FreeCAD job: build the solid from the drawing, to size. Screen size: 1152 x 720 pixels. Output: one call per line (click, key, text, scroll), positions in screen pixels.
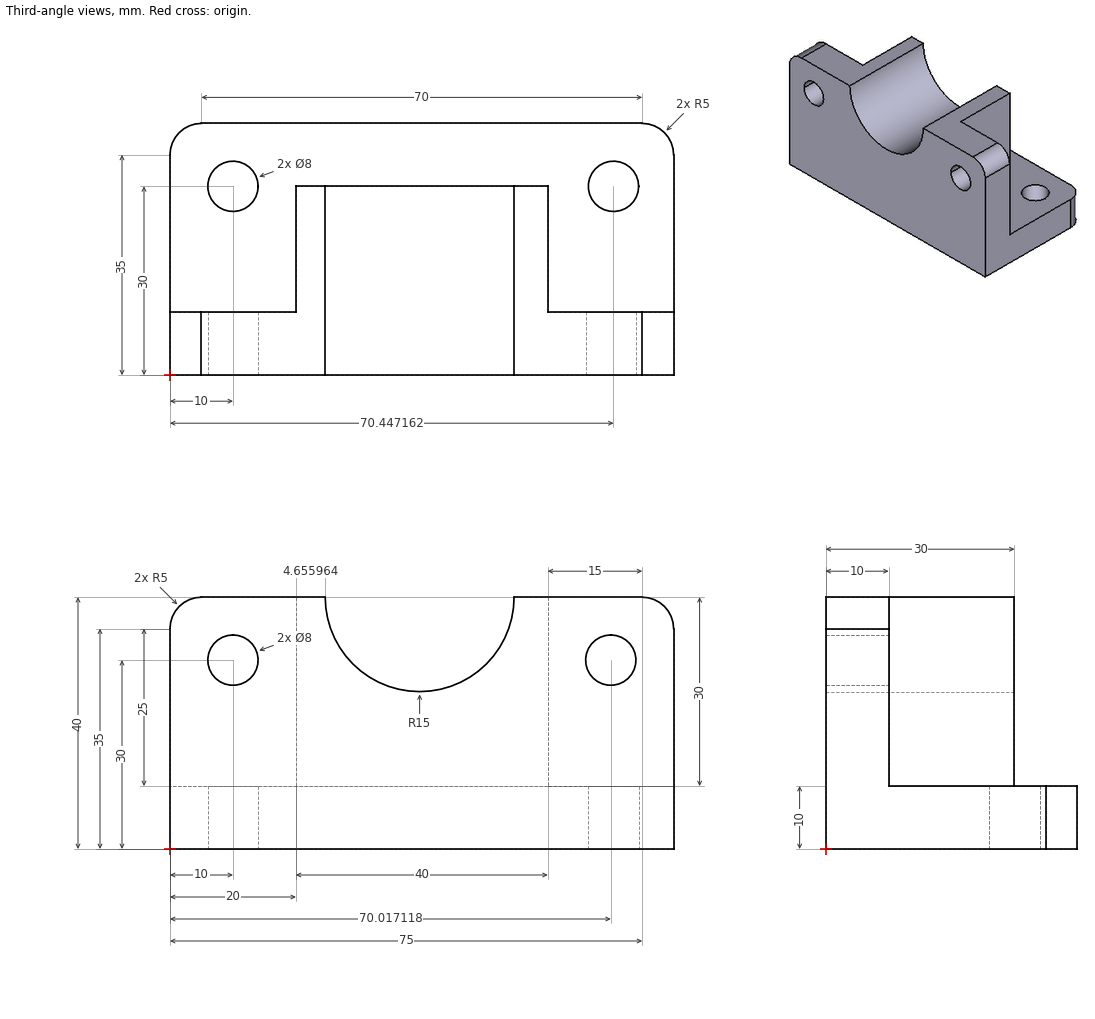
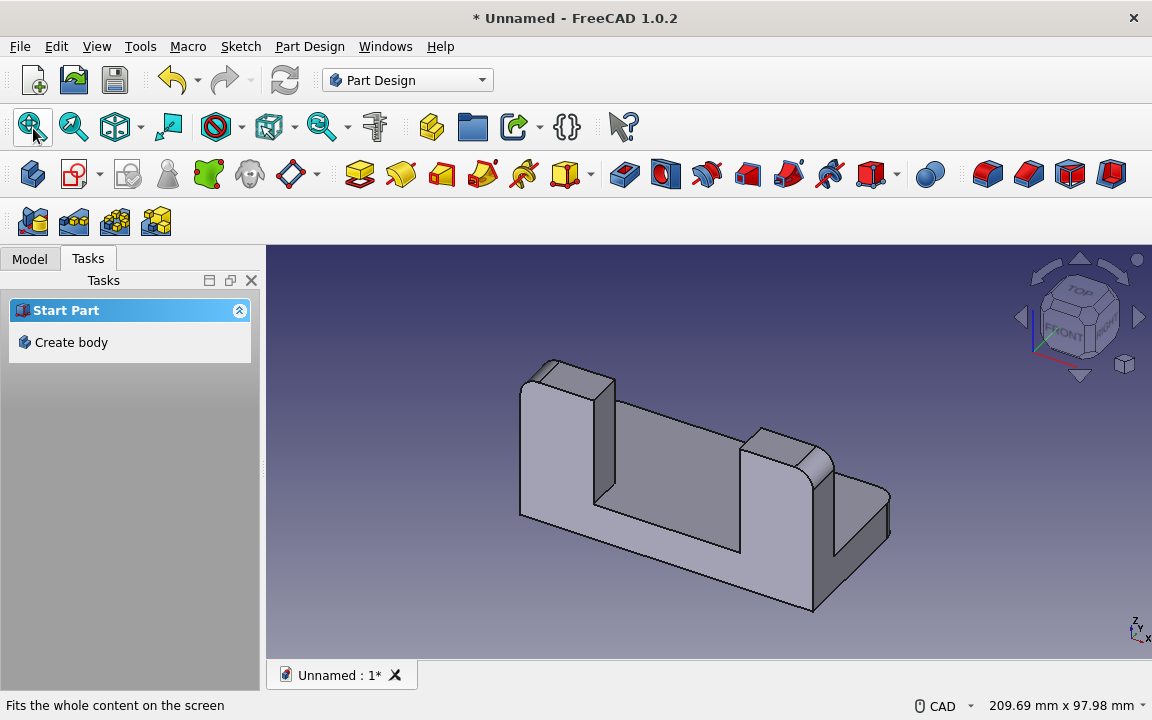
click(541, 412)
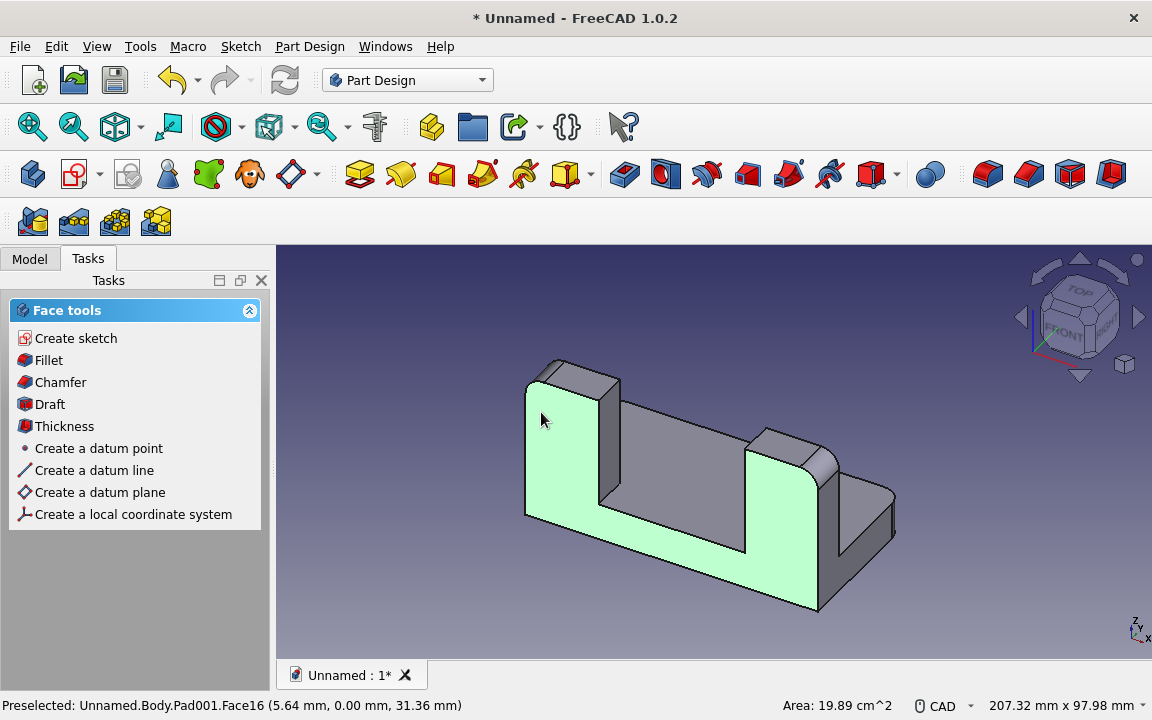
click(74, 174)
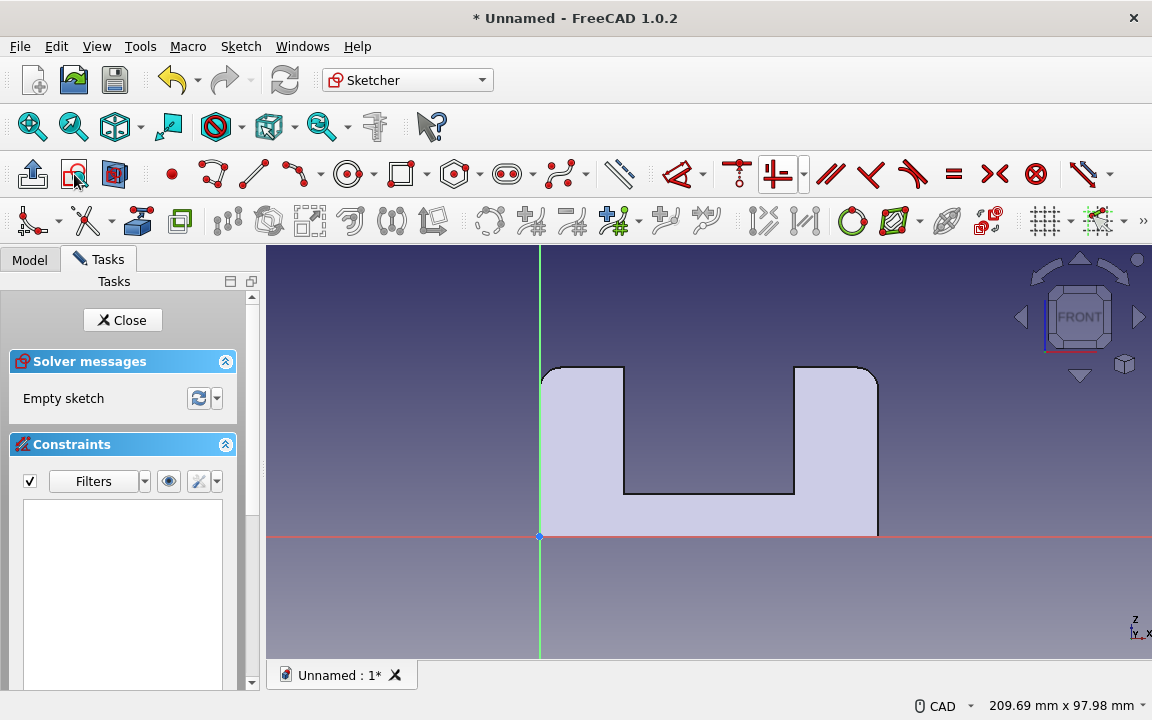
scroll(720, 452, up, 2)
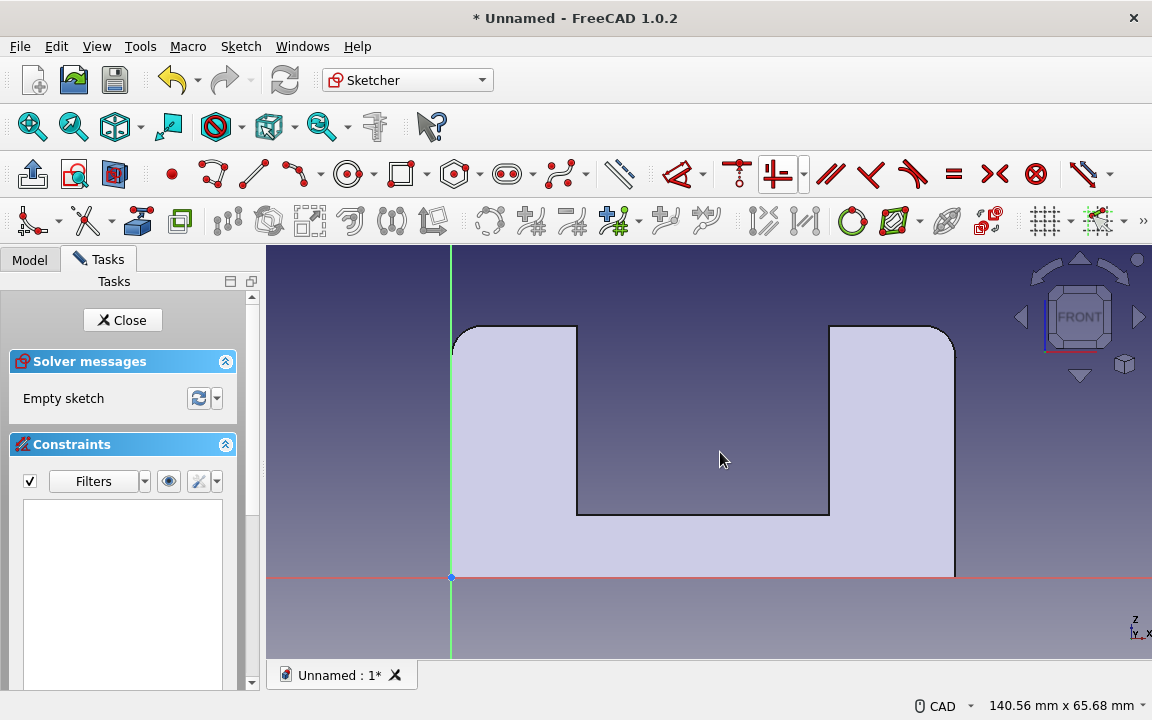
click(213, 174)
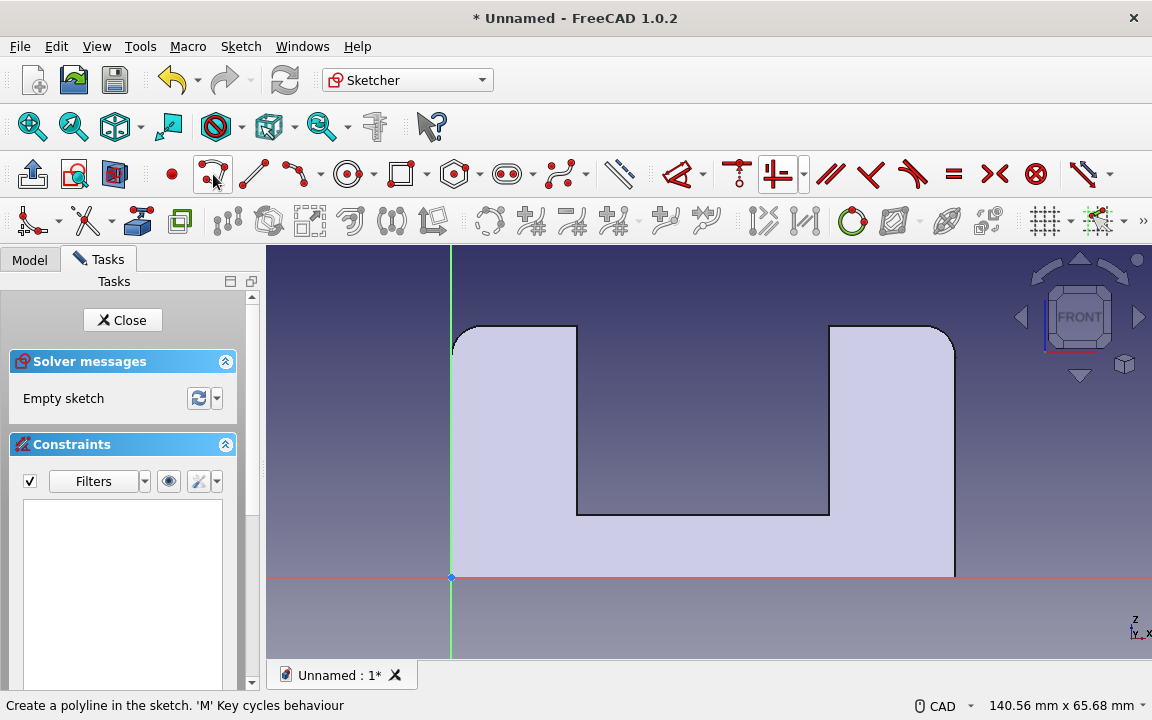
click(607, 326)
click(577, 326)
click(577, 515)
click(829, 515)
click(829, 326)
click(796, 326)
right_click(796, 326)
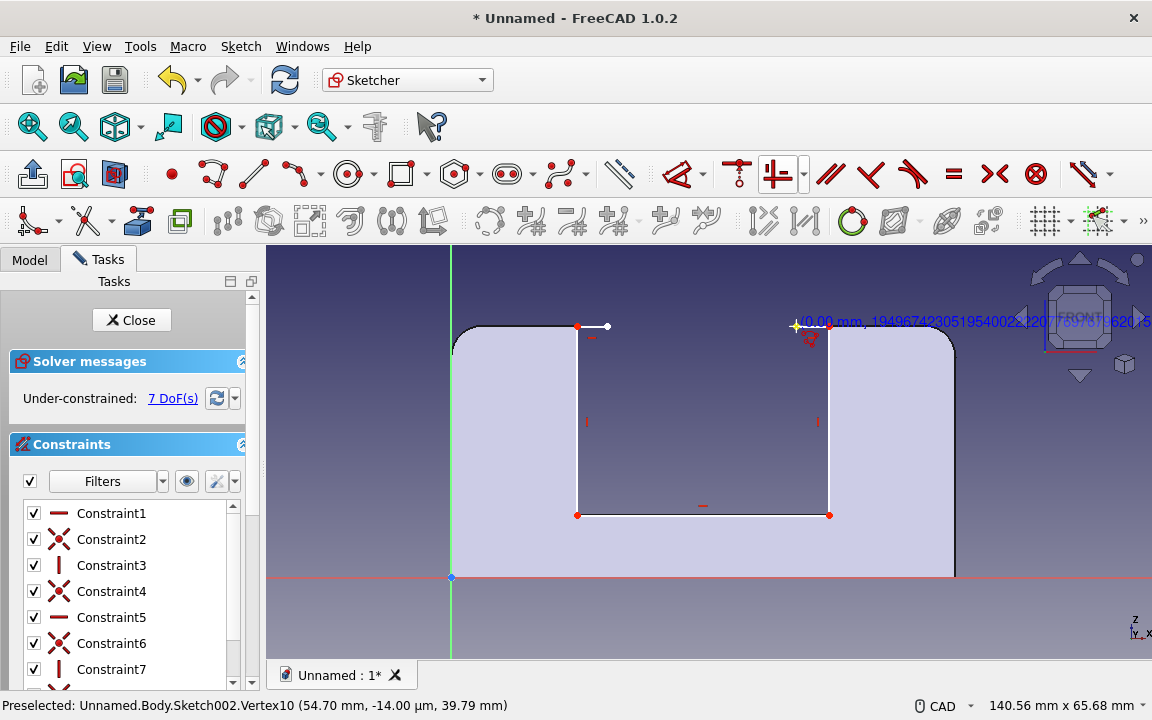
click(294, 174)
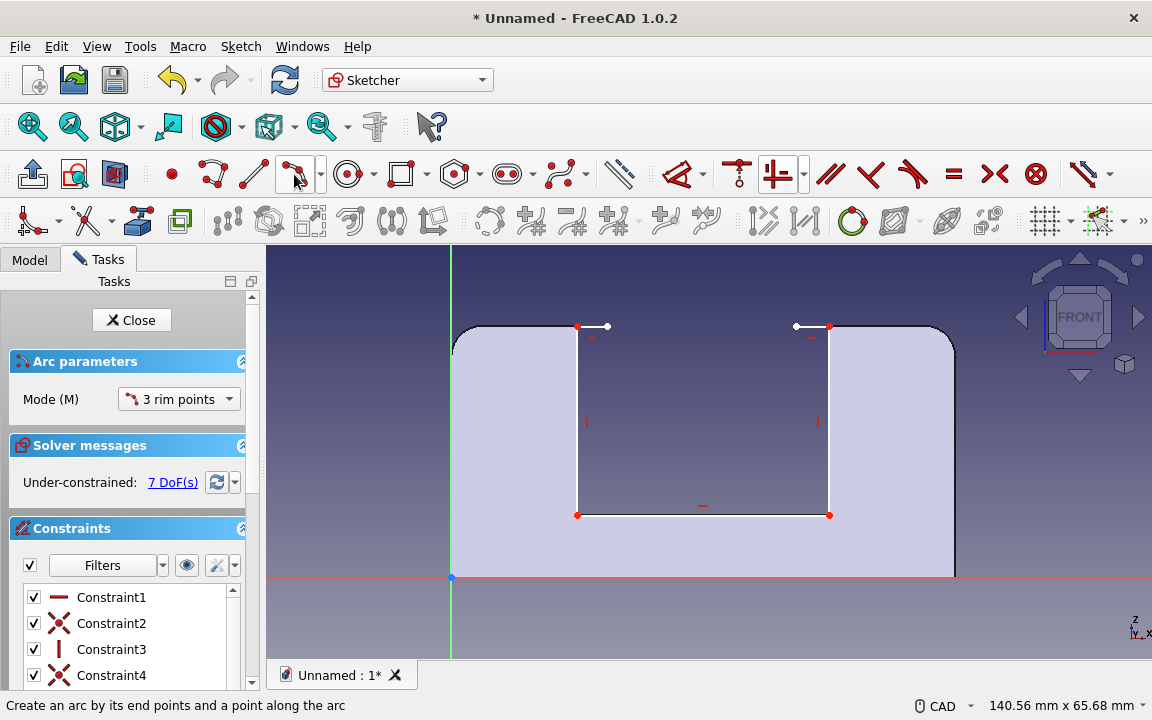
click(796, 327)
click(607, 327)
click(701, 420)
key(Escape)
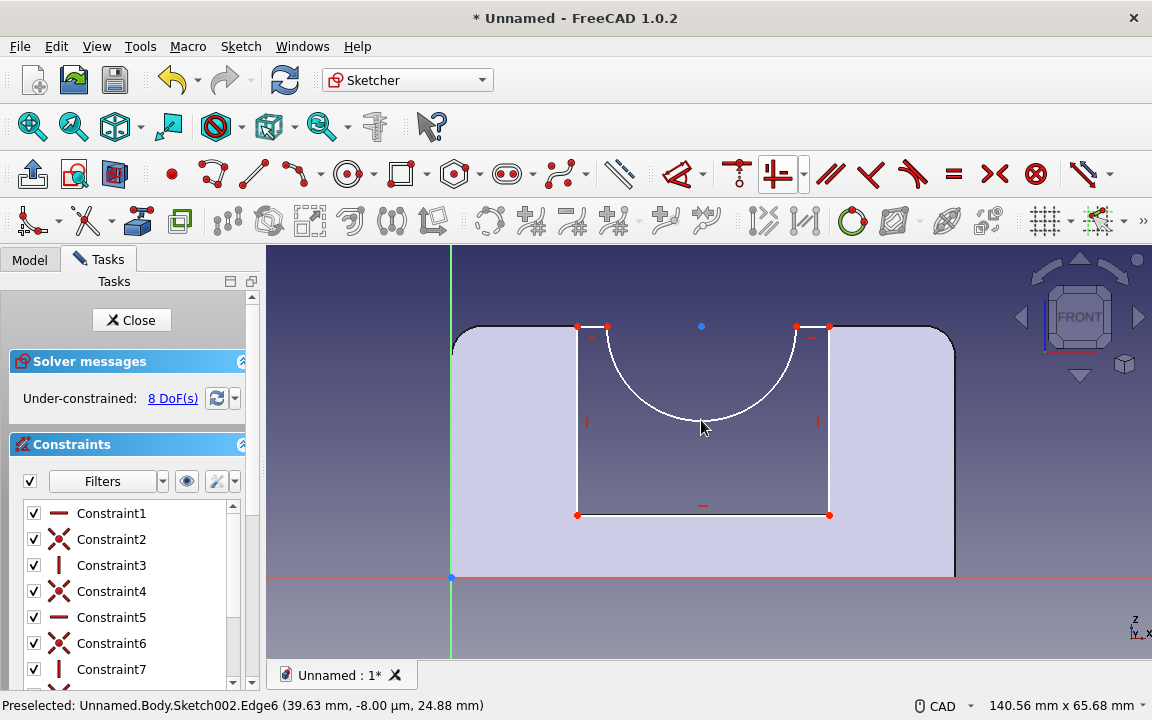
click(676, 174)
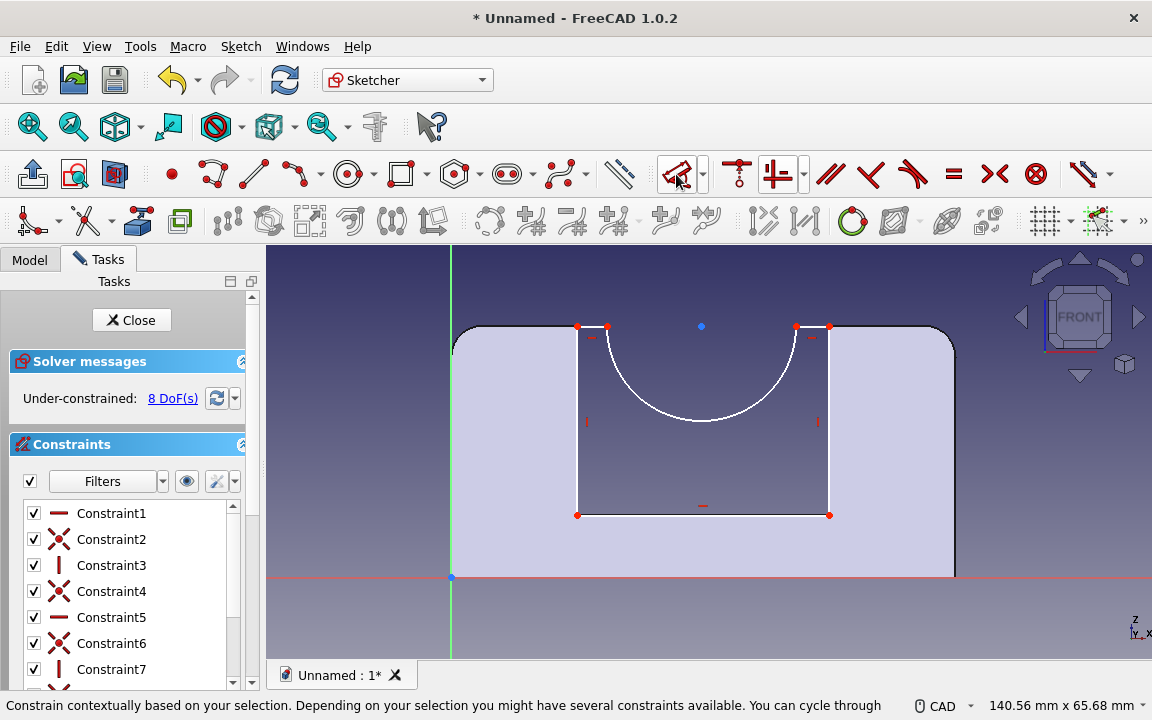
click(646, 403)
click(627, 429)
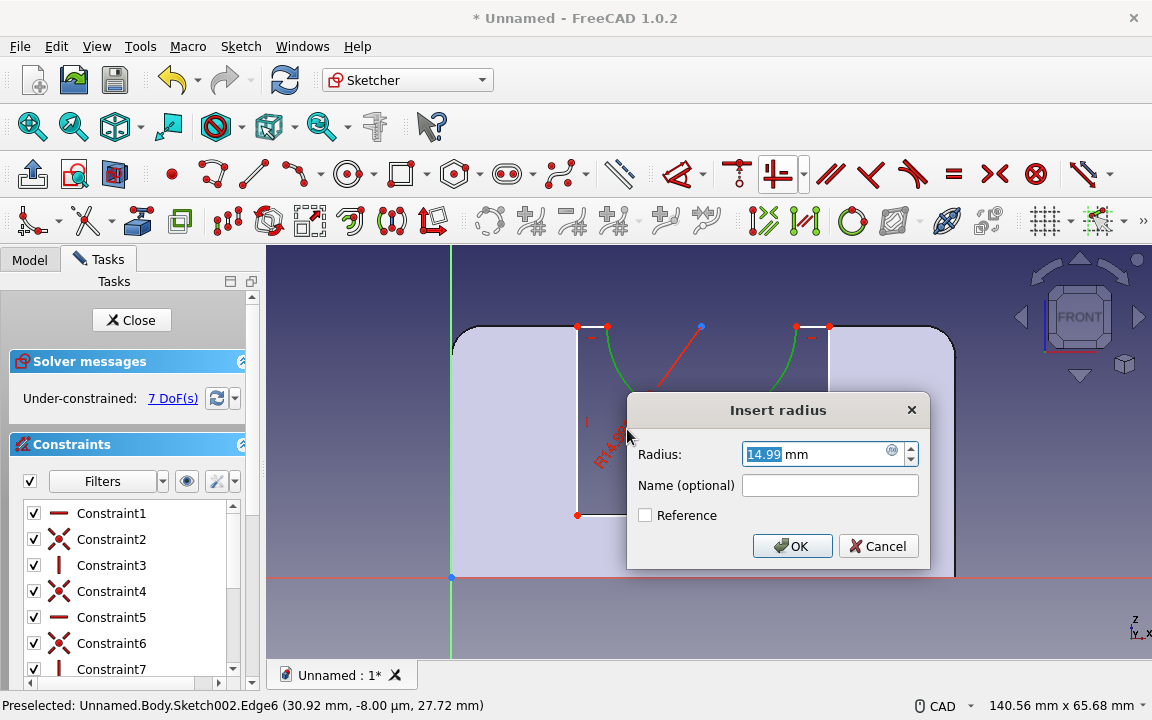
text(15)
key(Return)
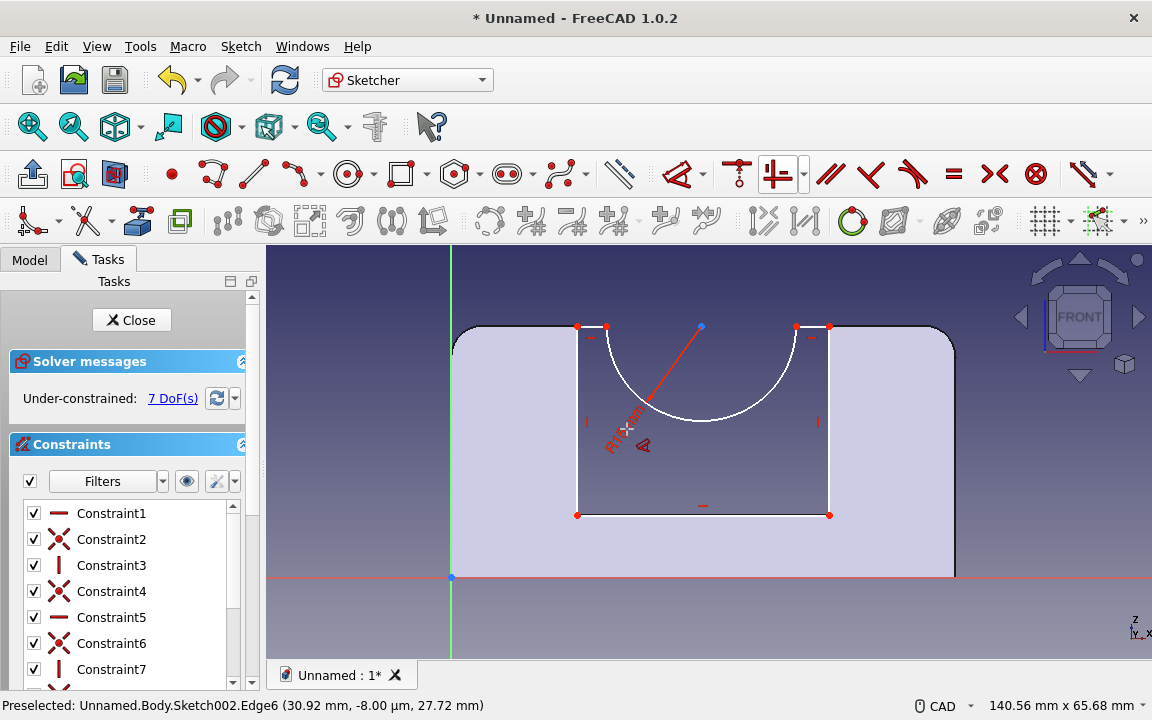
click(577, 384)
click(543, 421)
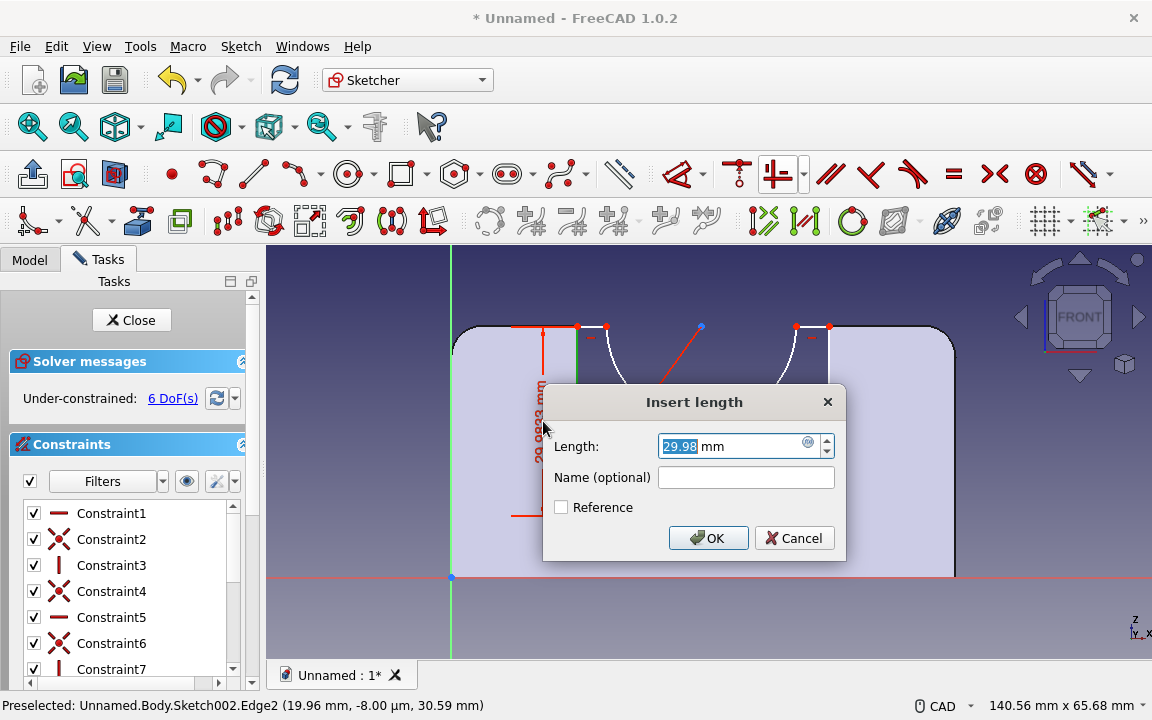
text(30)
key(Return)